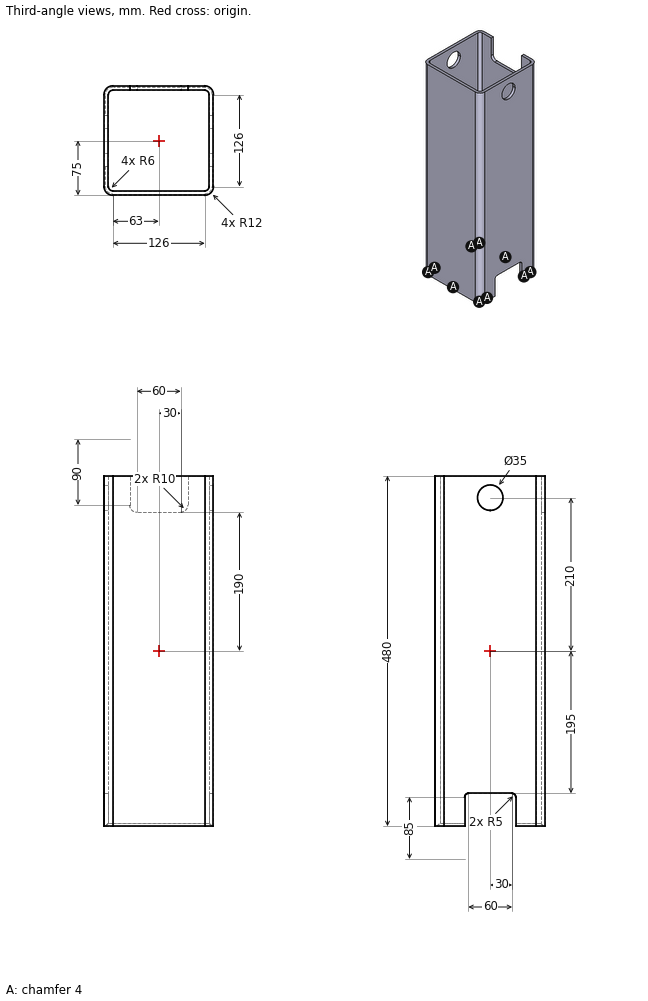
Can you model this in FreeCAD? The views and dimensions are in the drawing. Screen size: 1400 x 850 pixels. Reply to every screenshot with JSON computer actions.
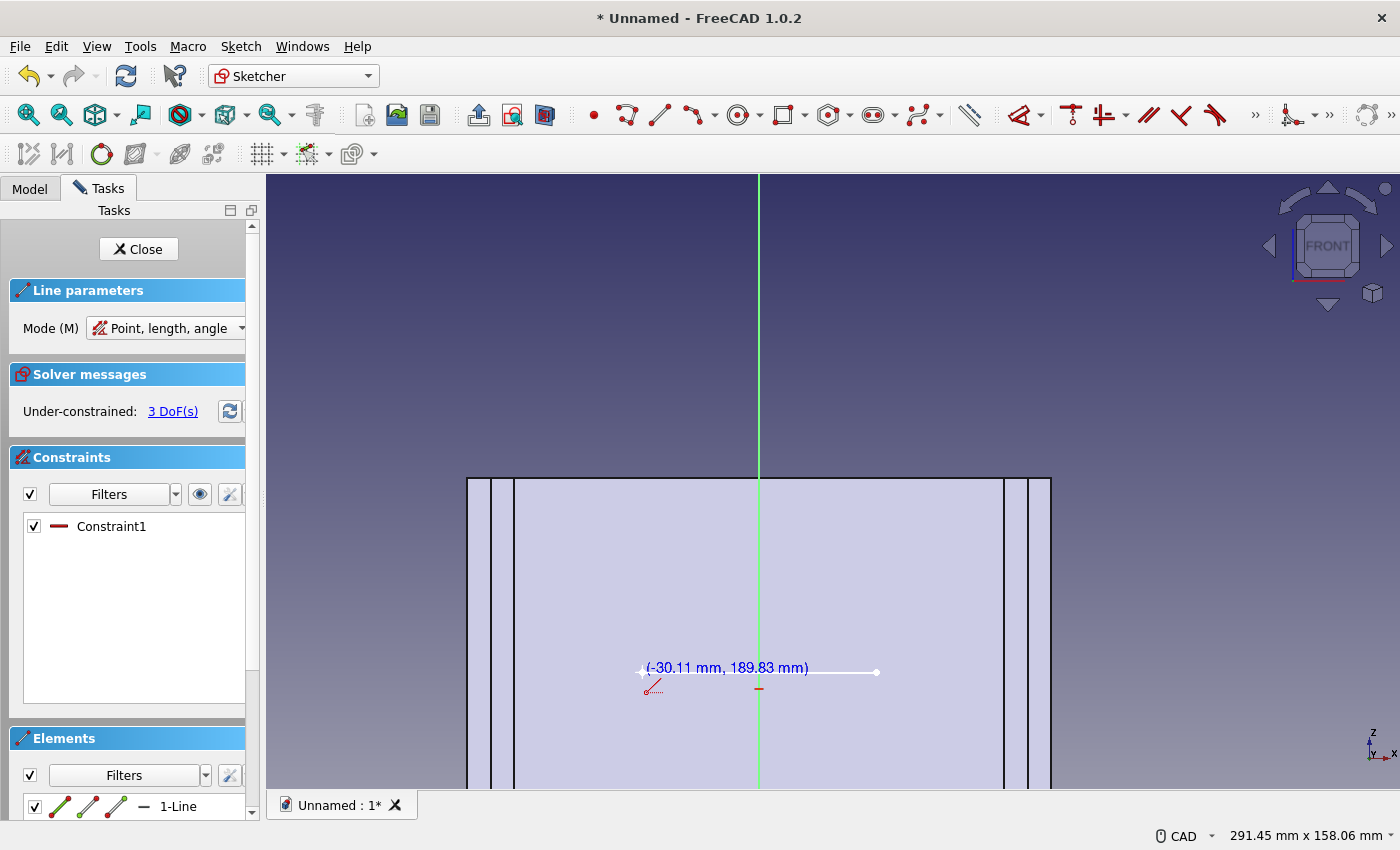
{"action": "key", "text": "g m"}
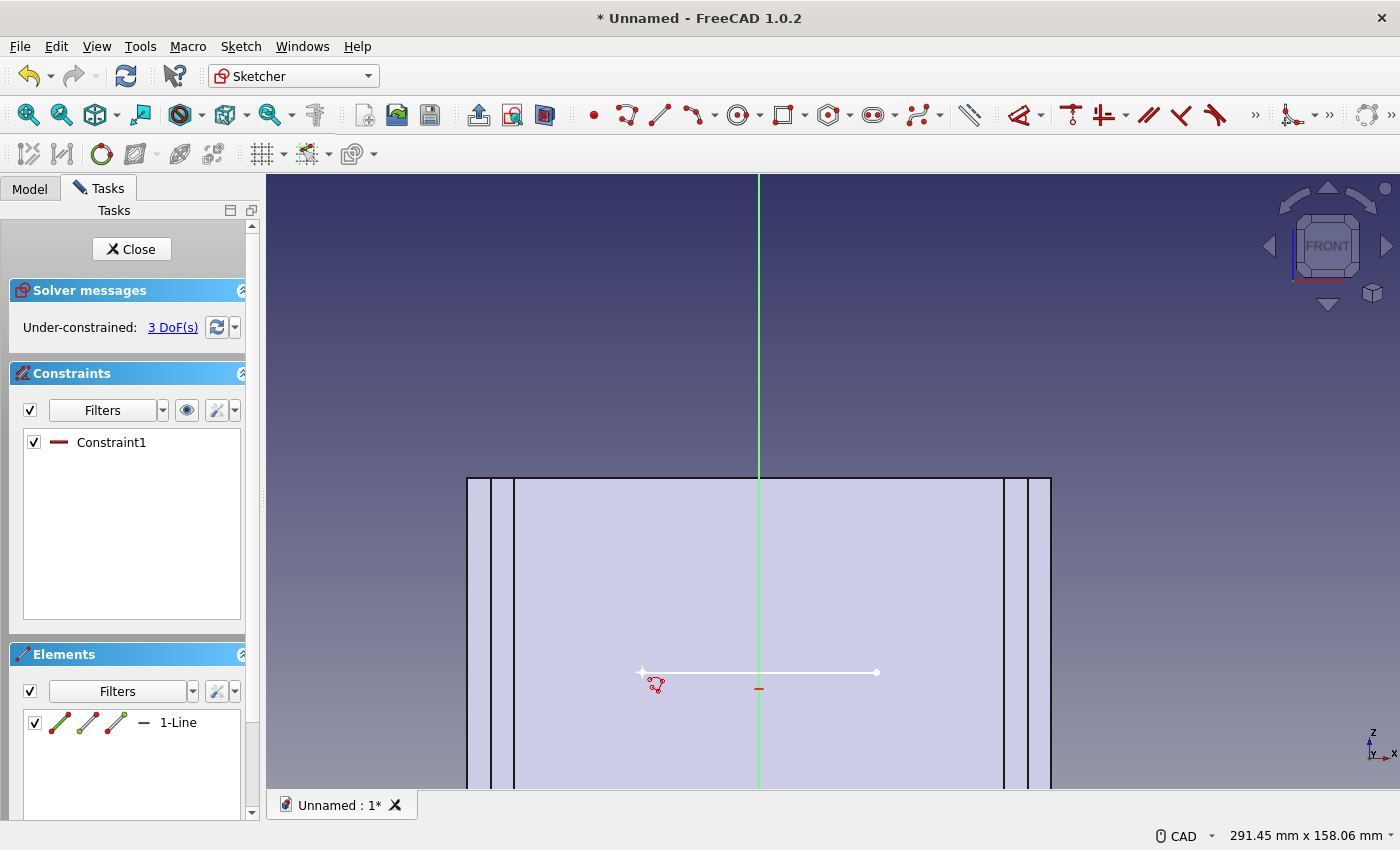
{"action": "left_click", "coordinate": [604, 633]}
{"action": "left_click", "coordinate": [604, 283]}
{"action": "left_click", "coordinate": [915, 283]}
{"action": "left_click", "coordinate": [915, 633]}
{"action": "right_click", "coordinate": [915, 633]}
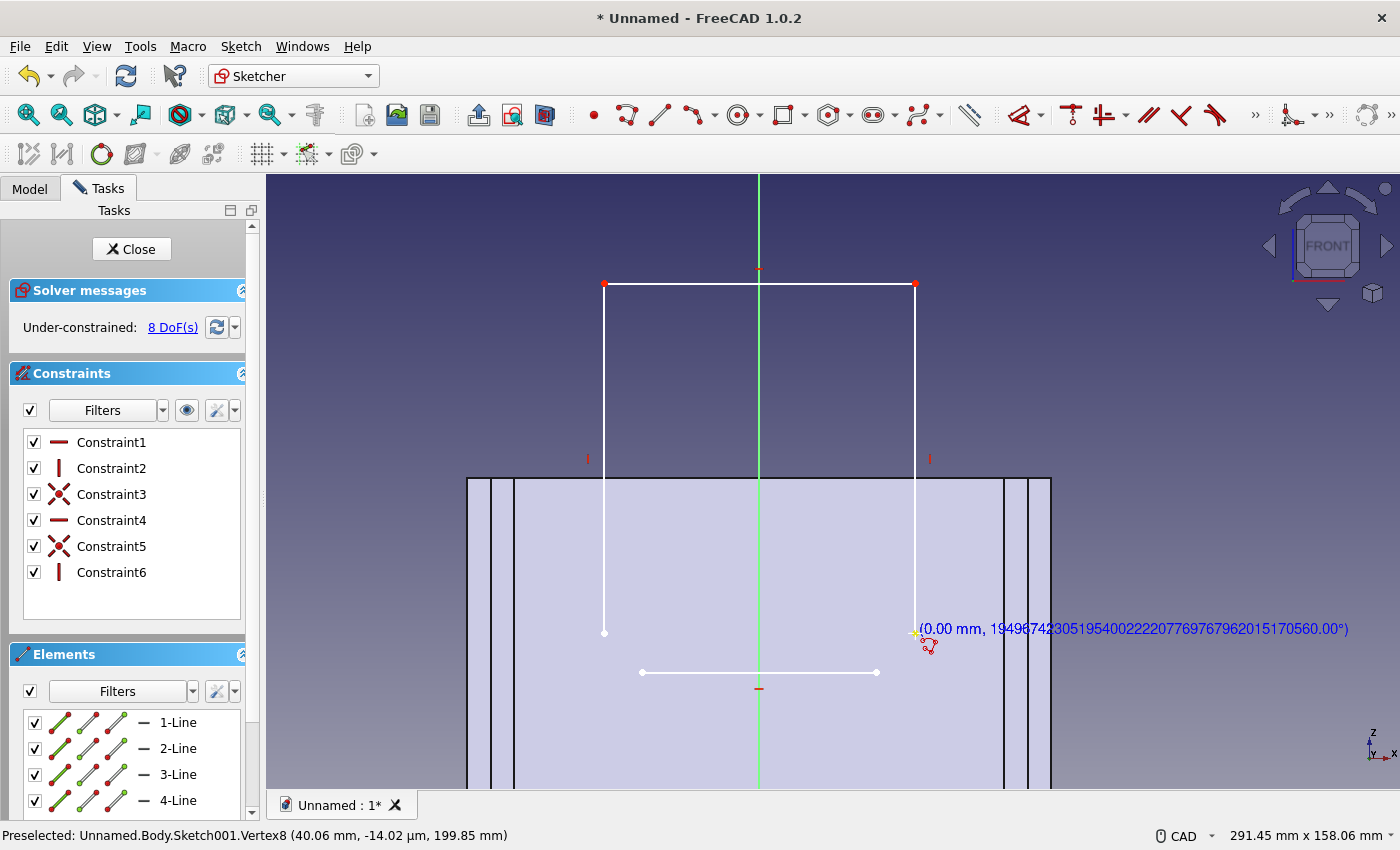
{"action": "key", "text": "g 3 a"}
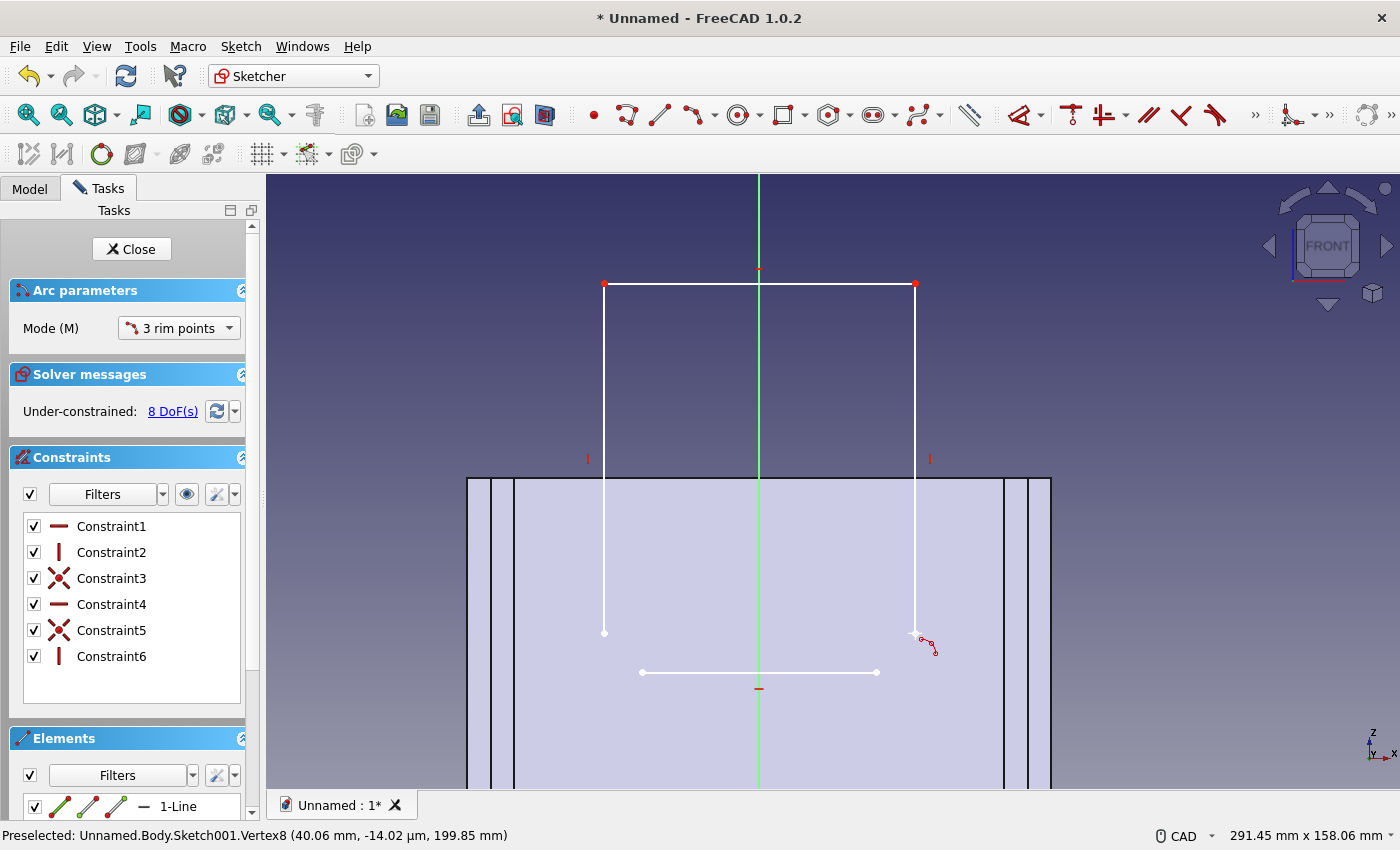
{"action": "left_click", "coordinate": [642, 673]}
{"action": "left_click", "coordinate": [604, 634]}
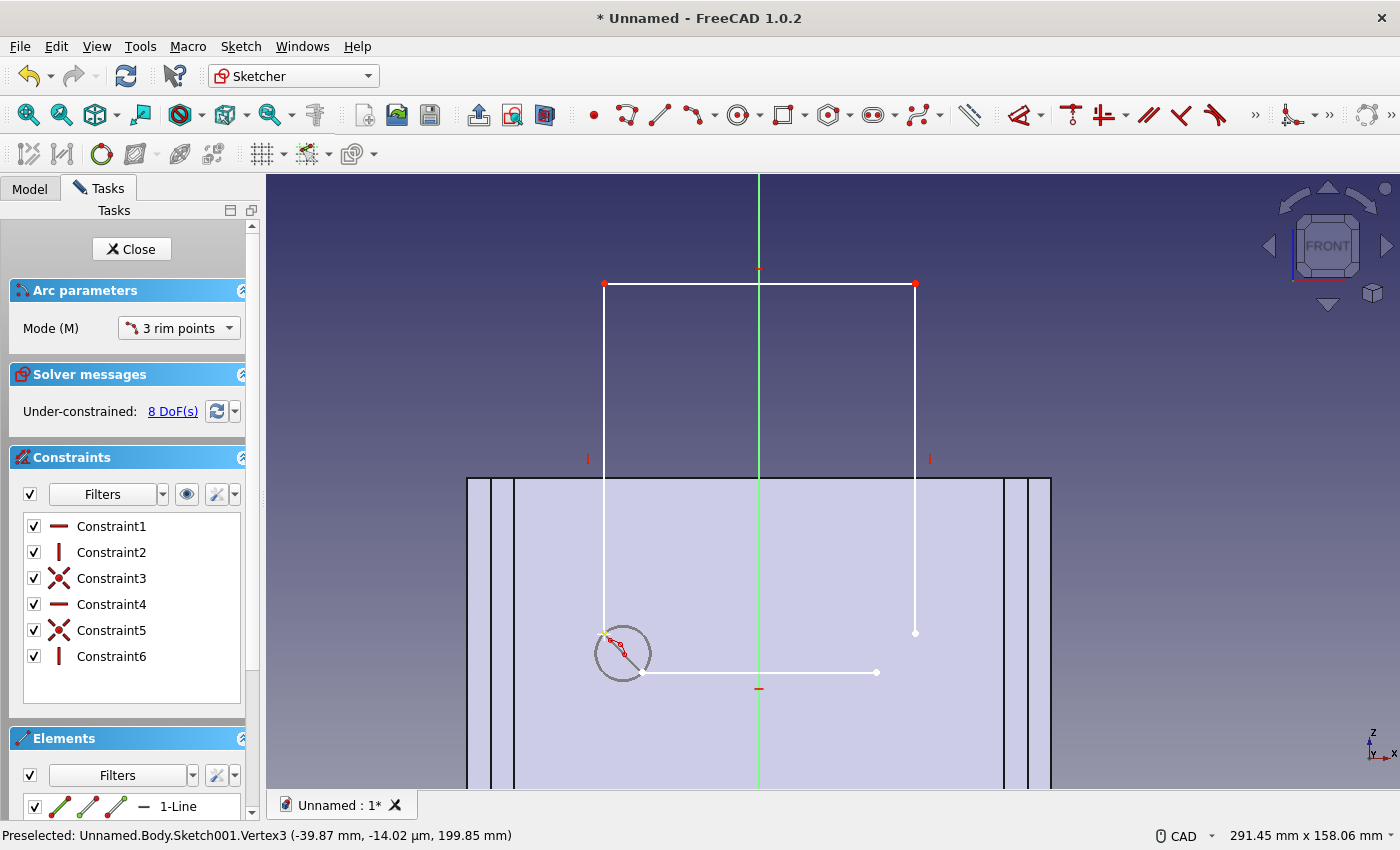
{"action": "scroll", "coordinate": [615, 661], "scroll_direction": "up", "scroll_amount": 2}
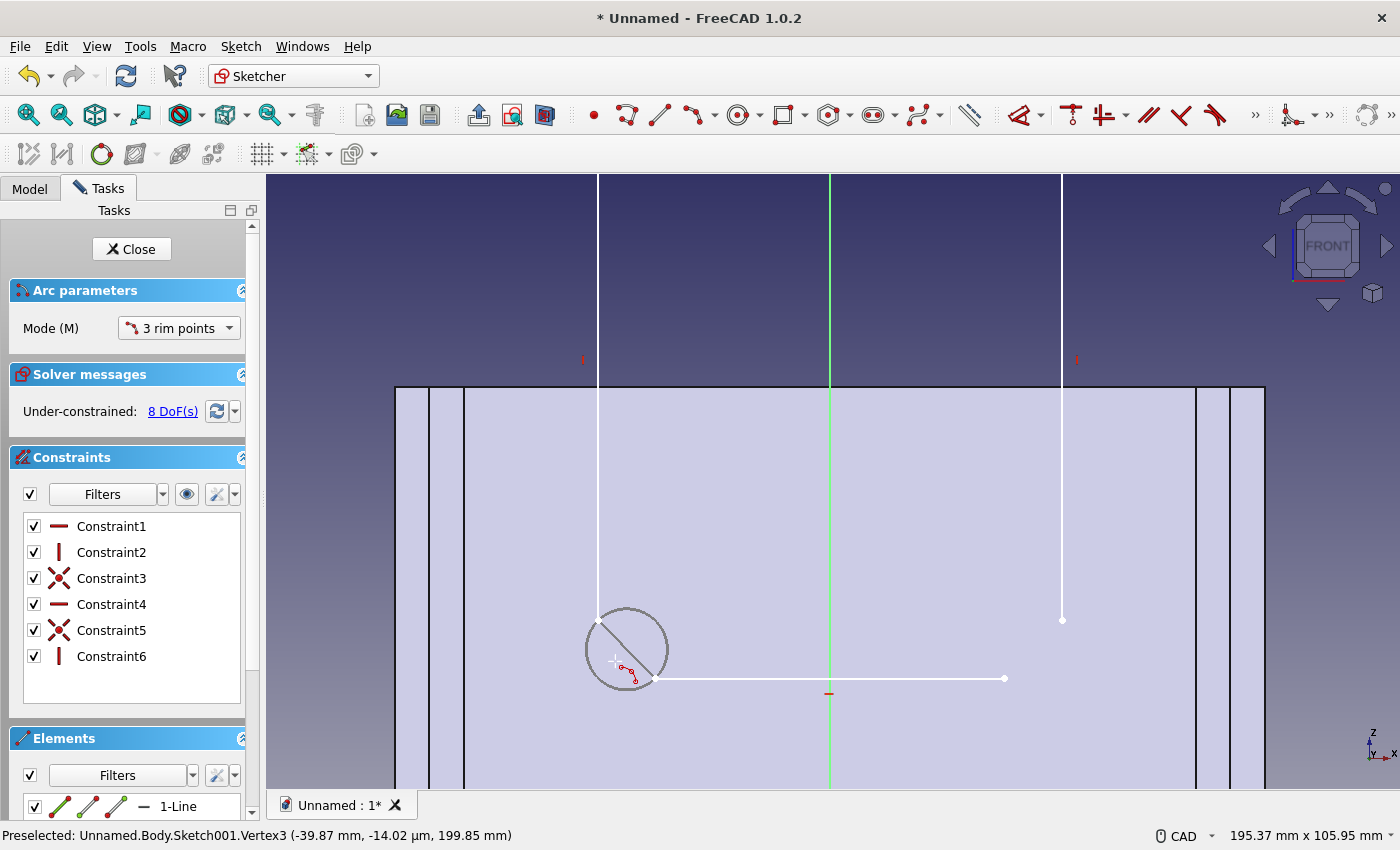
{"action": "left_click", "coordinate": [615, 661]}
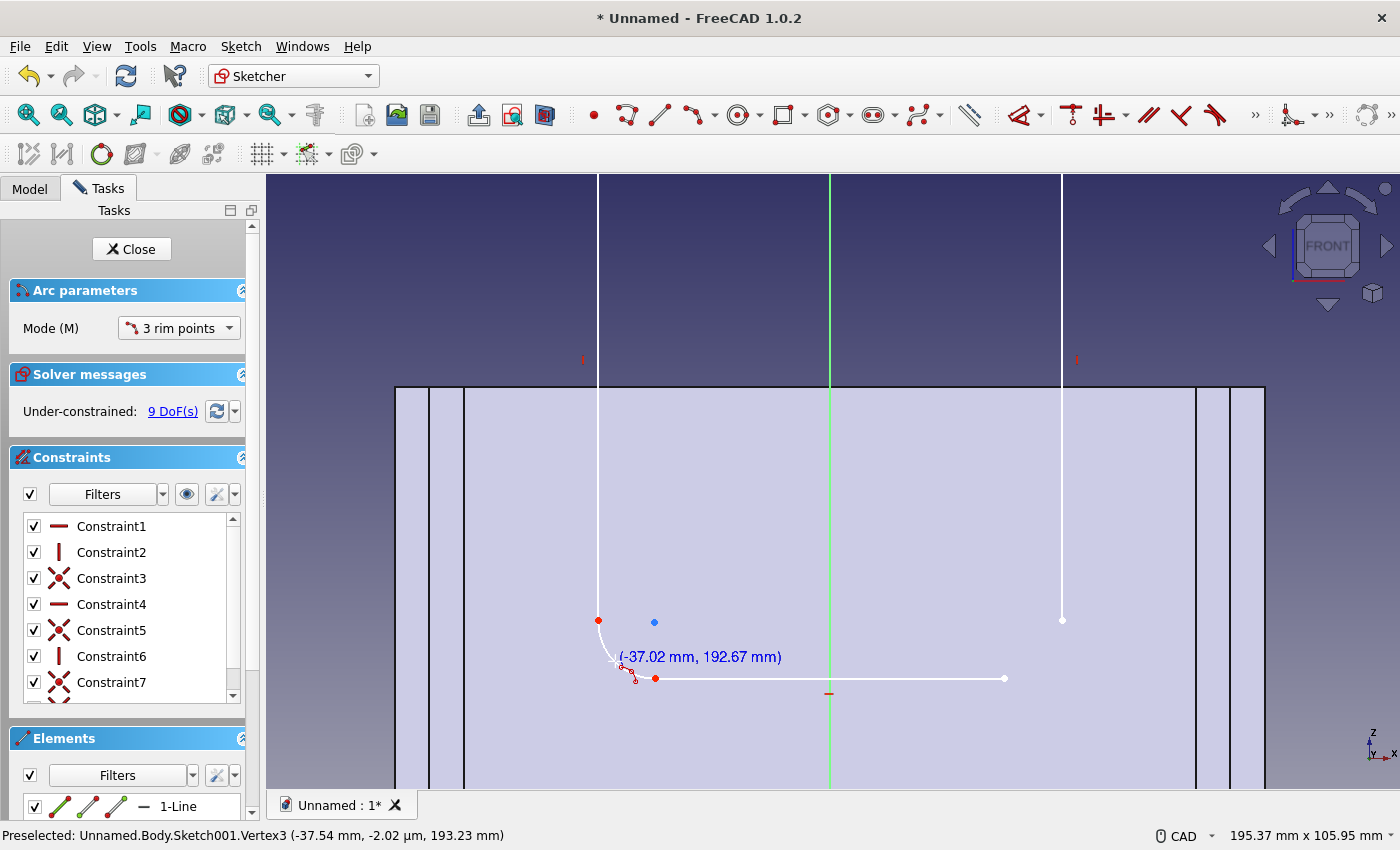
{"action": "left_click", "coordinate": [1062, 620]}
{"action": "left_click", "coordinate": [1004, 679]}
{"action": "left_click", "coordinate": [1045, 661]}
{"action": "key", "text": "Escape"}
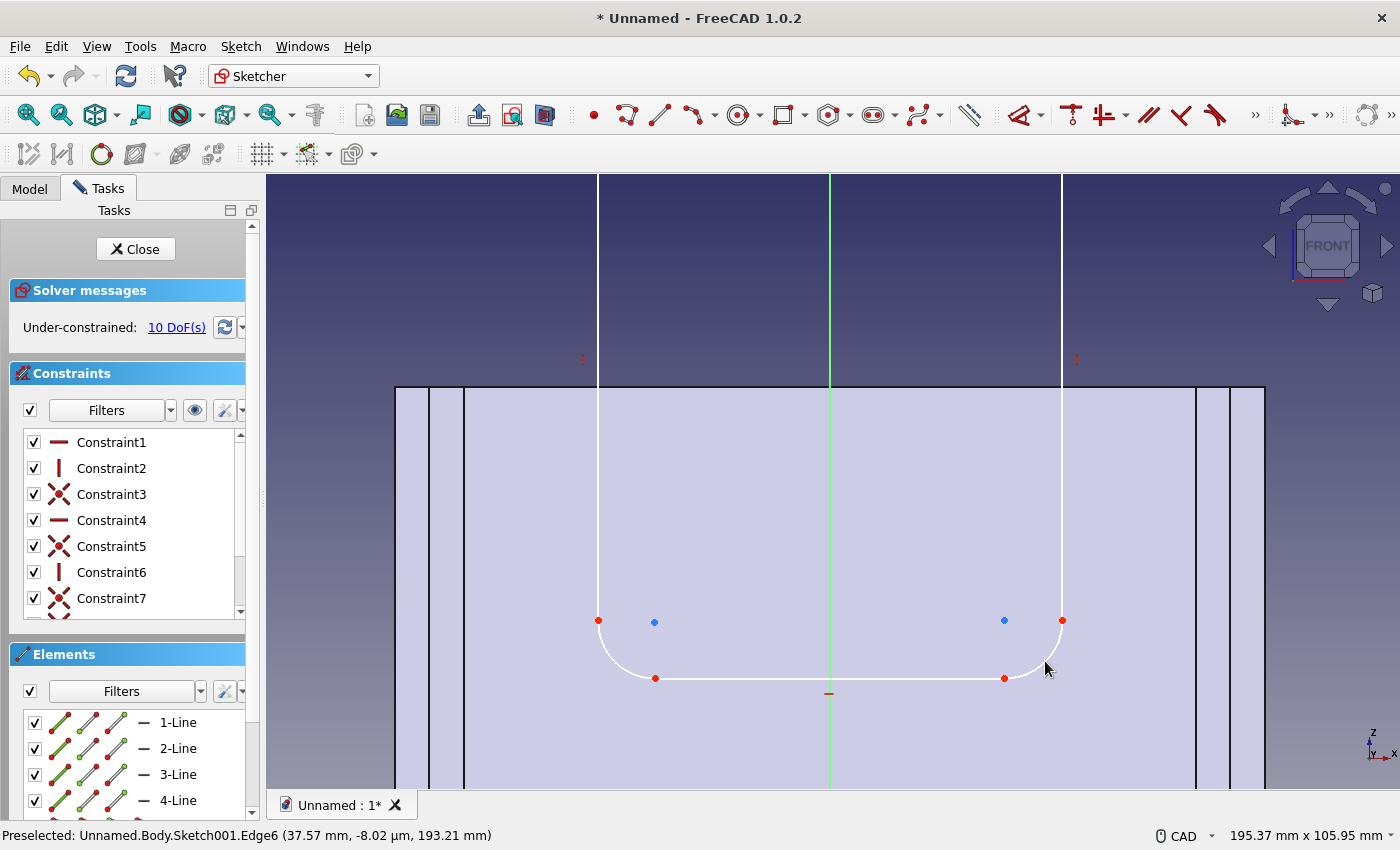
{"action": "left_click", "coordinate": [899, 679]}